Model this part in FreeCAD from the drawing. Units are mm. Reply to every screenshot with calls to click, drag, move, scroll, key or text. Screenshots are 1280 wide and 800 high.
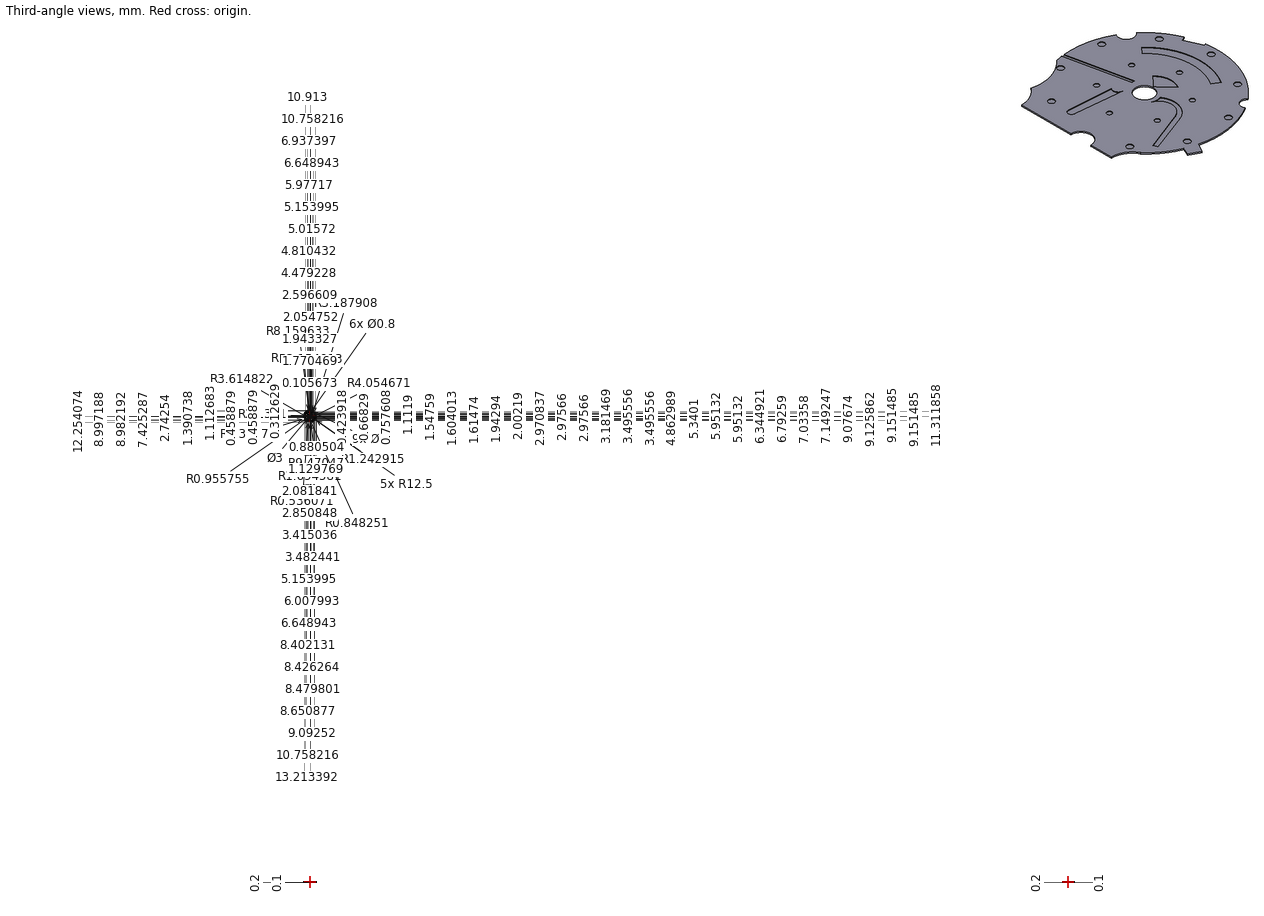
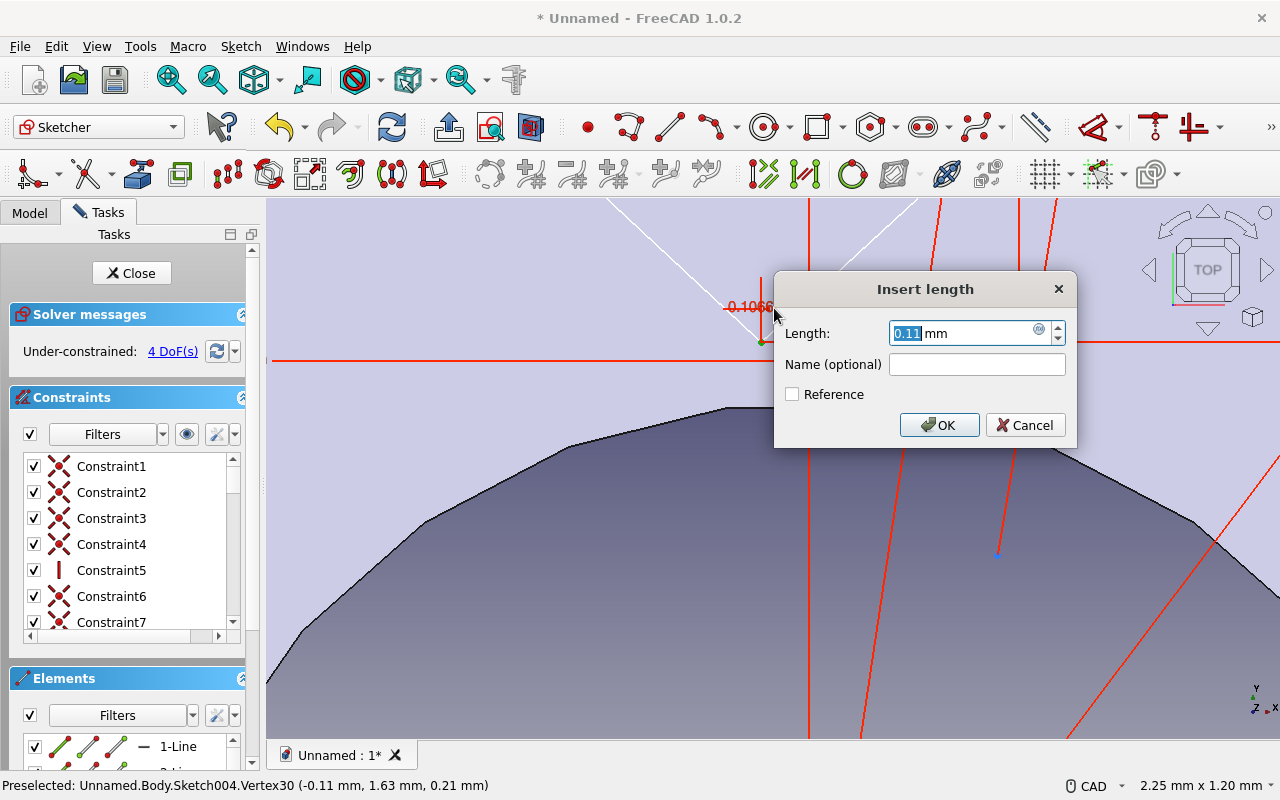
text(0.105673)
key(Return)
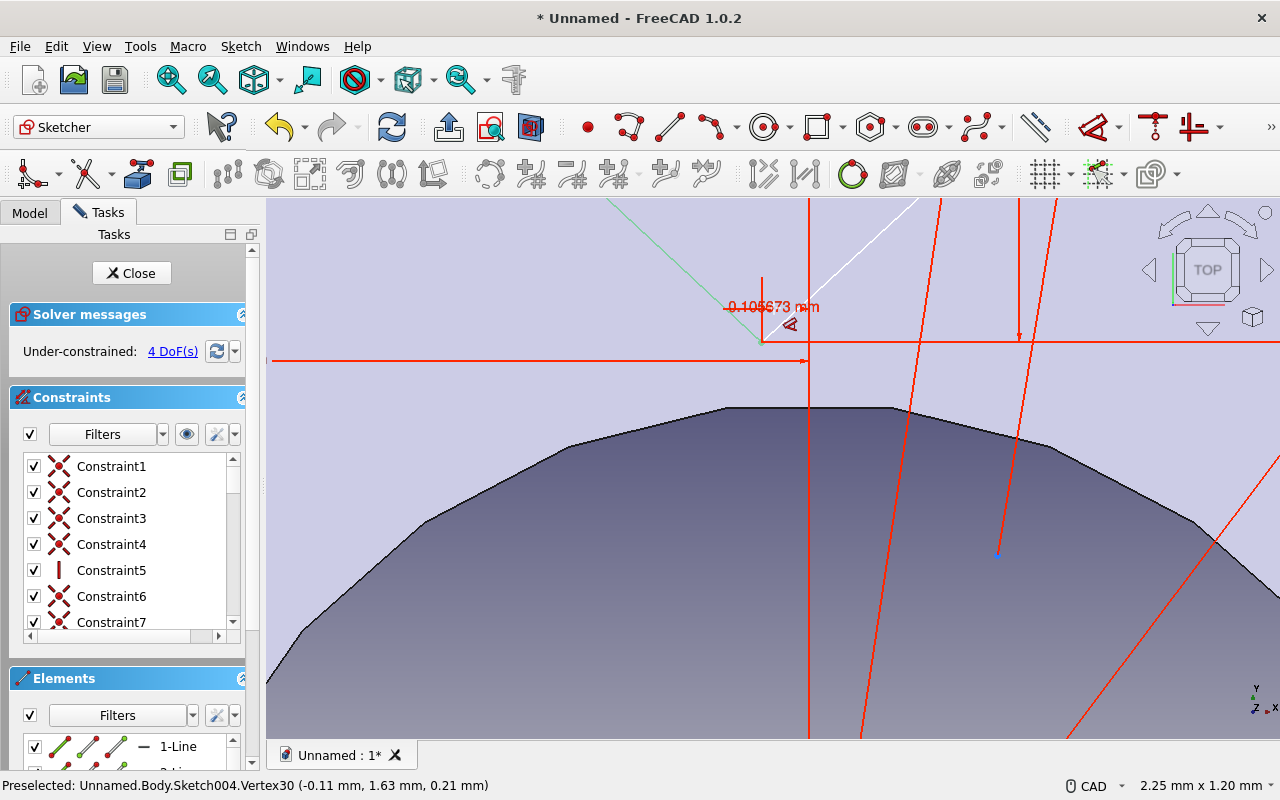
scroll(748, 434, down, 15)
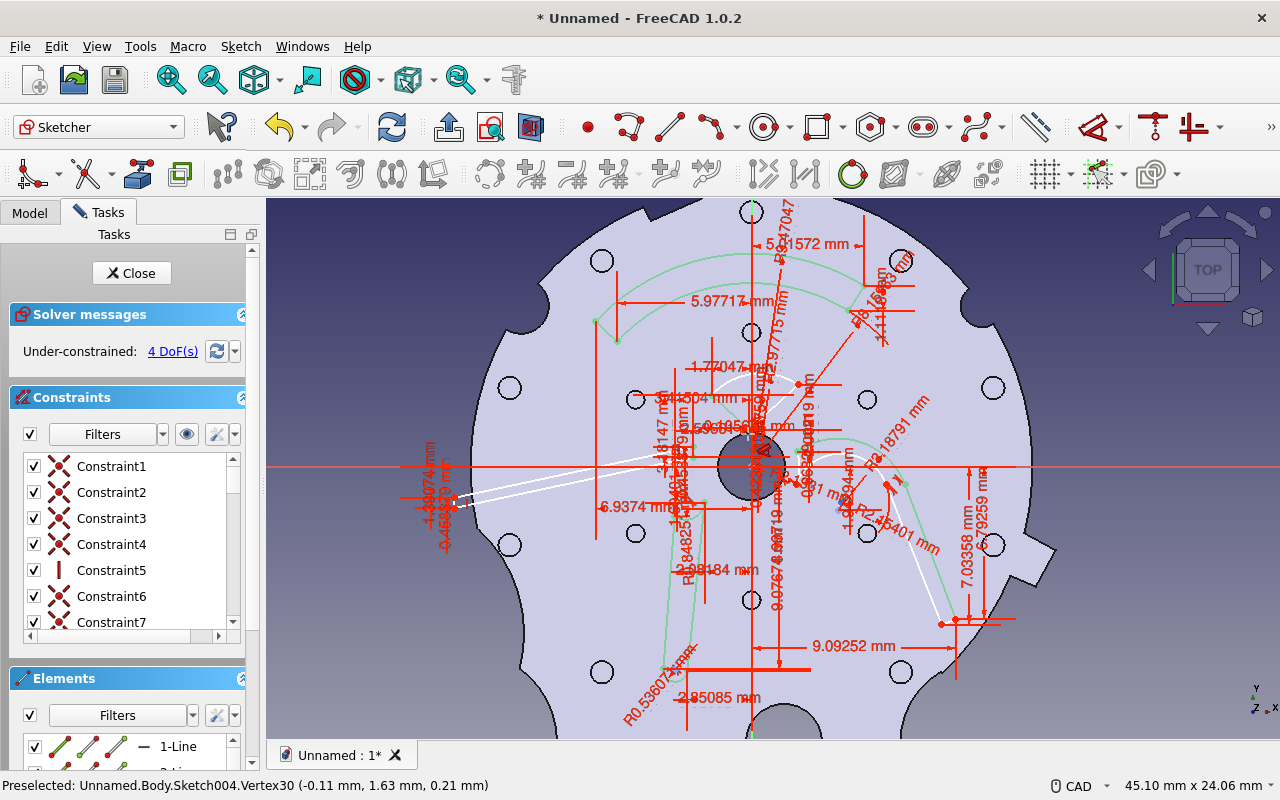
click(798, 385)
click(775, 549)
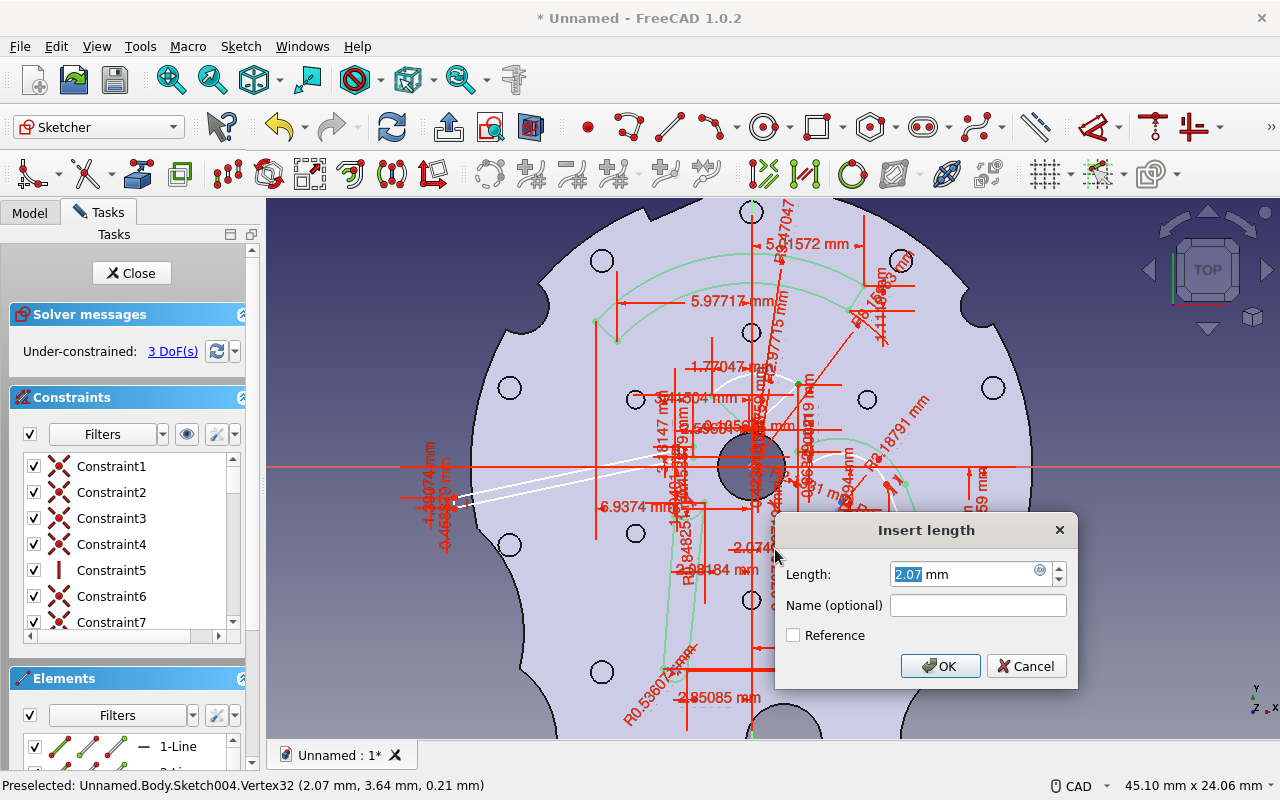
text(2.054752)
key(Return)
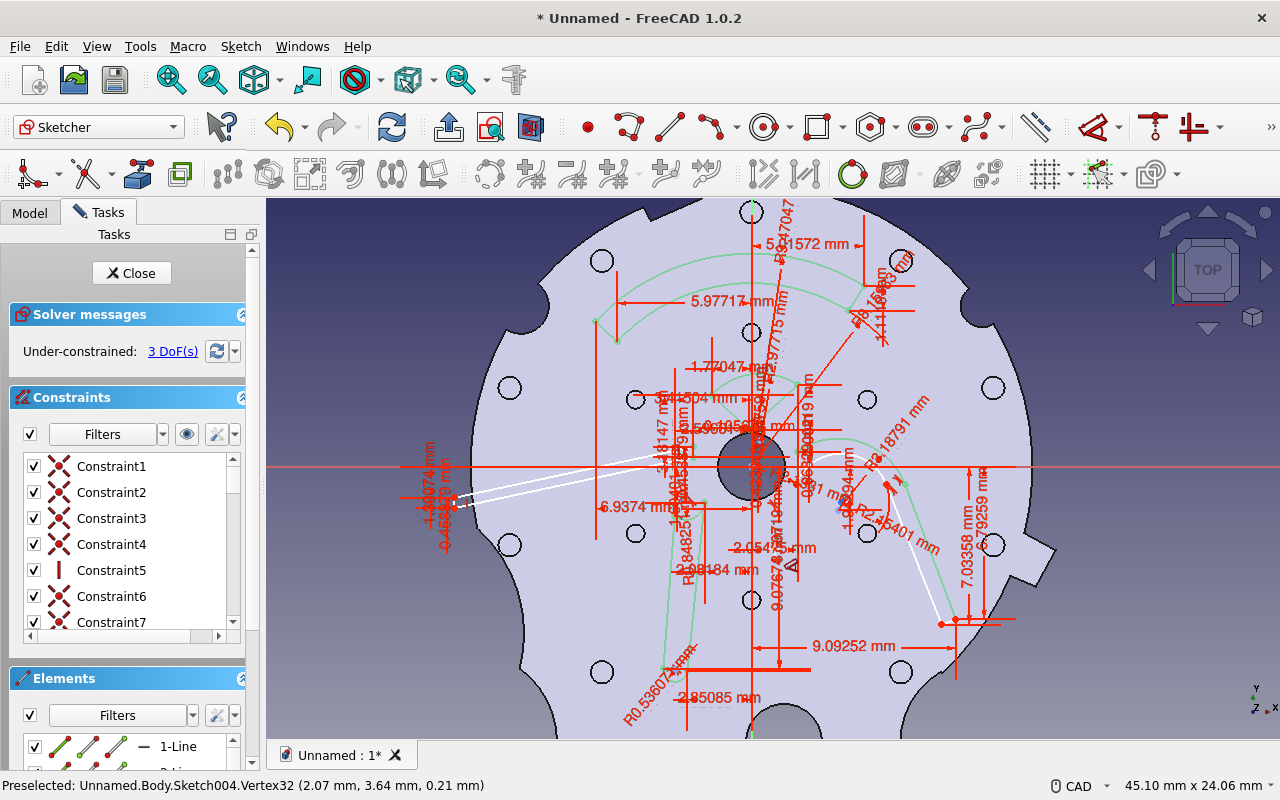
click(886, 484)
click(850, 566)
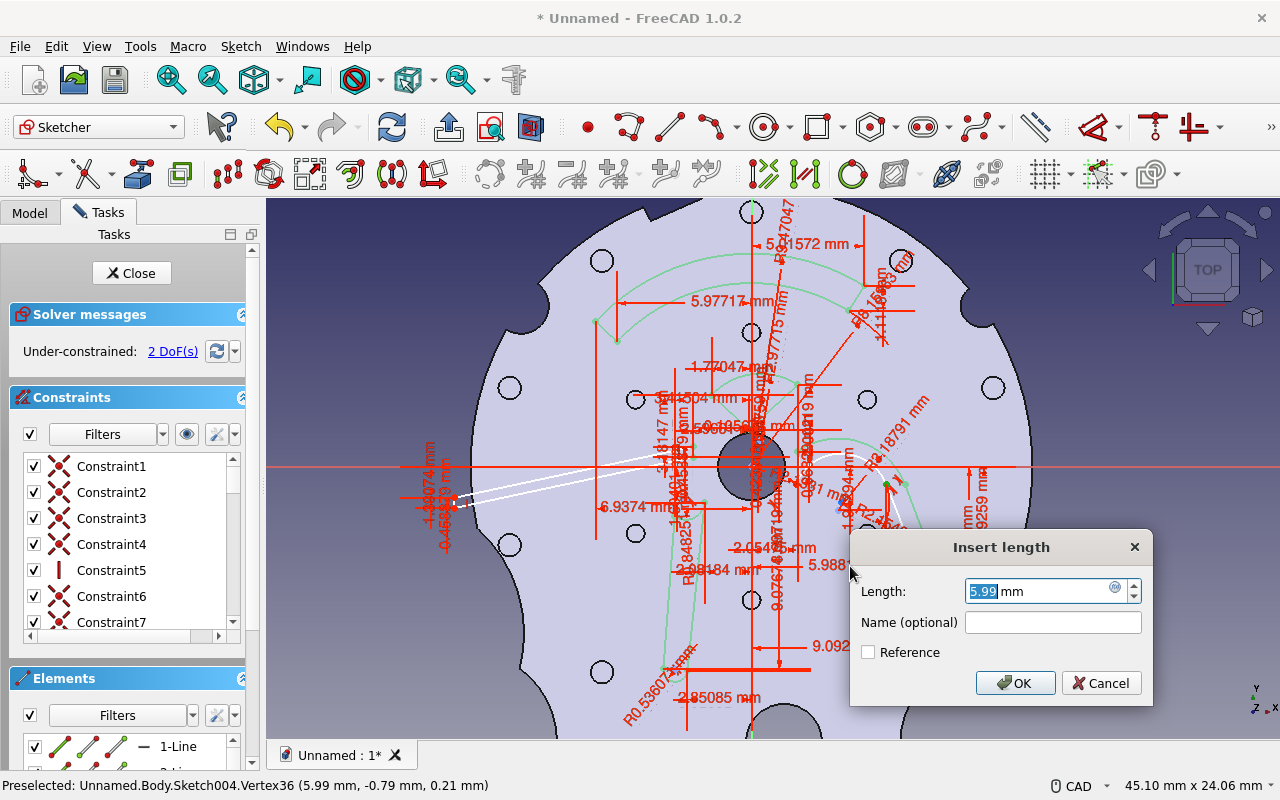
text(6.007993)
key(Return)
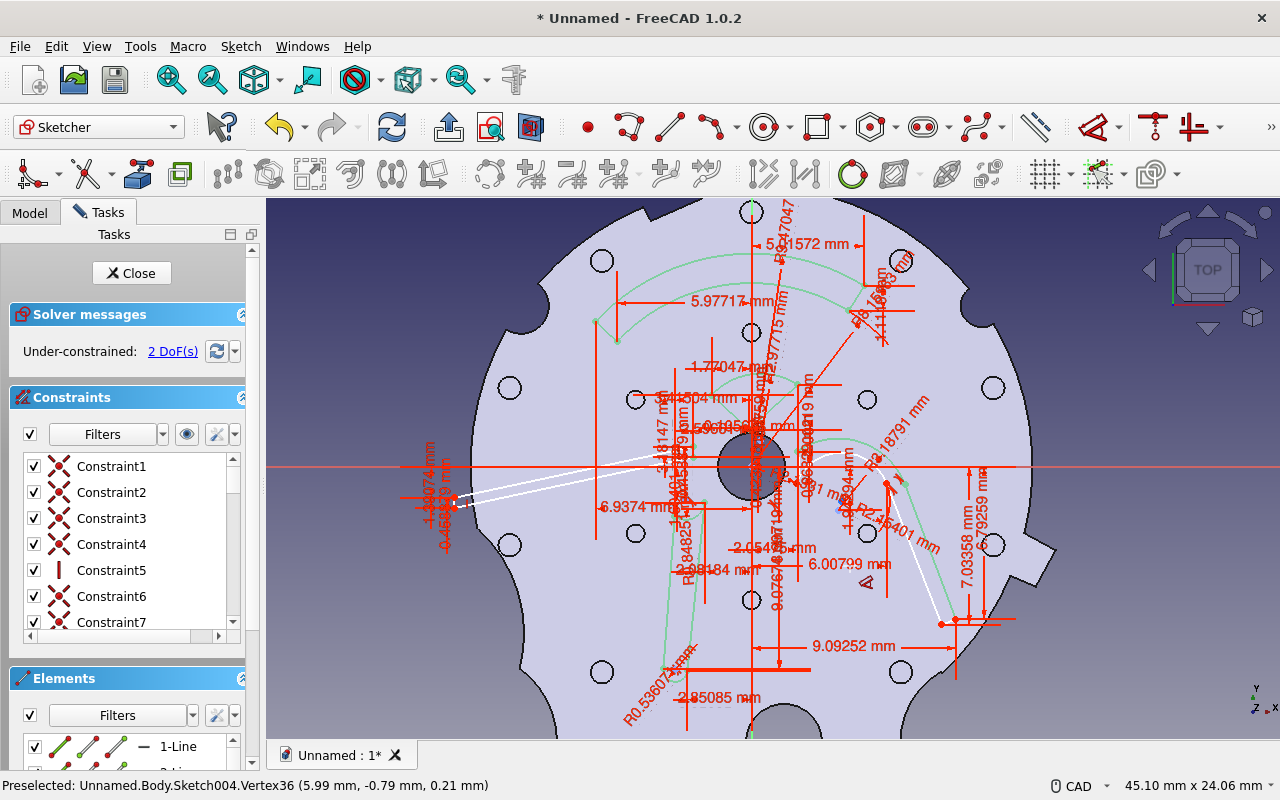
scroll(887, 484, up, 5)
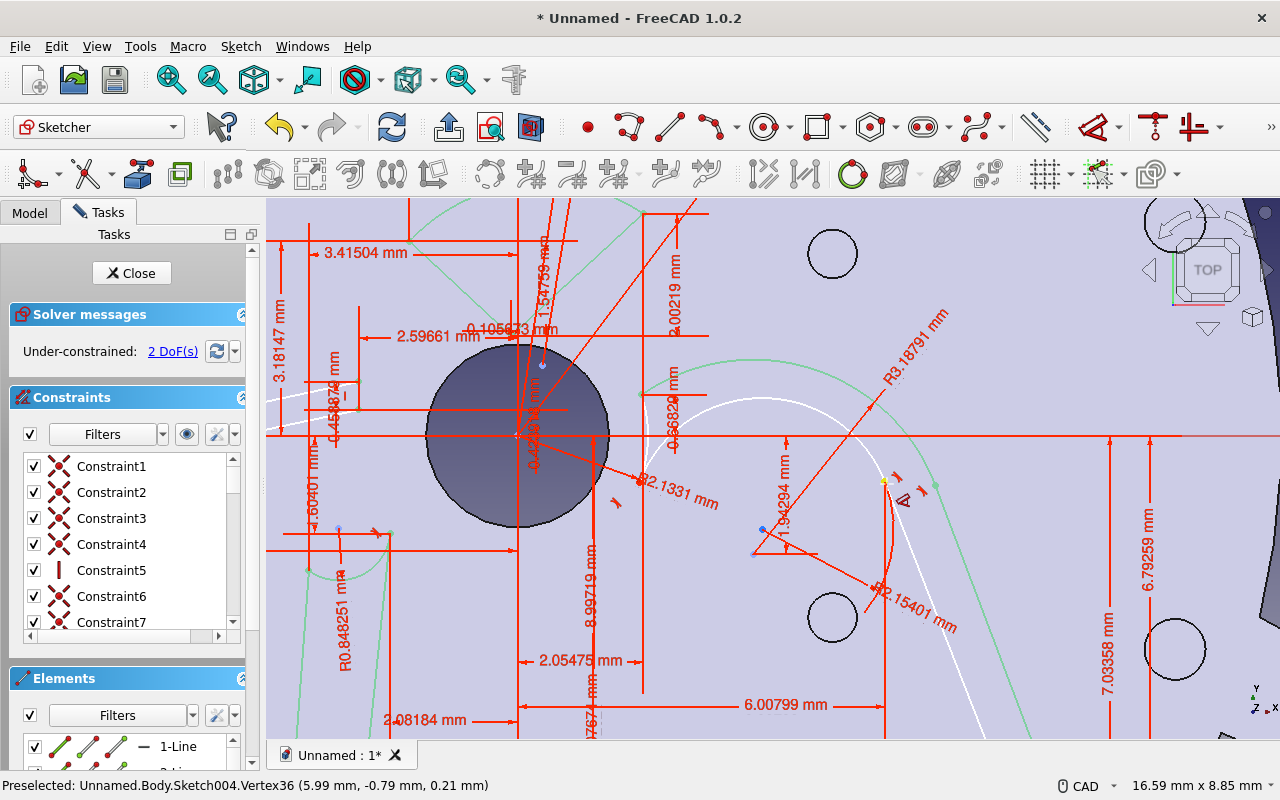
click(885, 482)
click(484, 459)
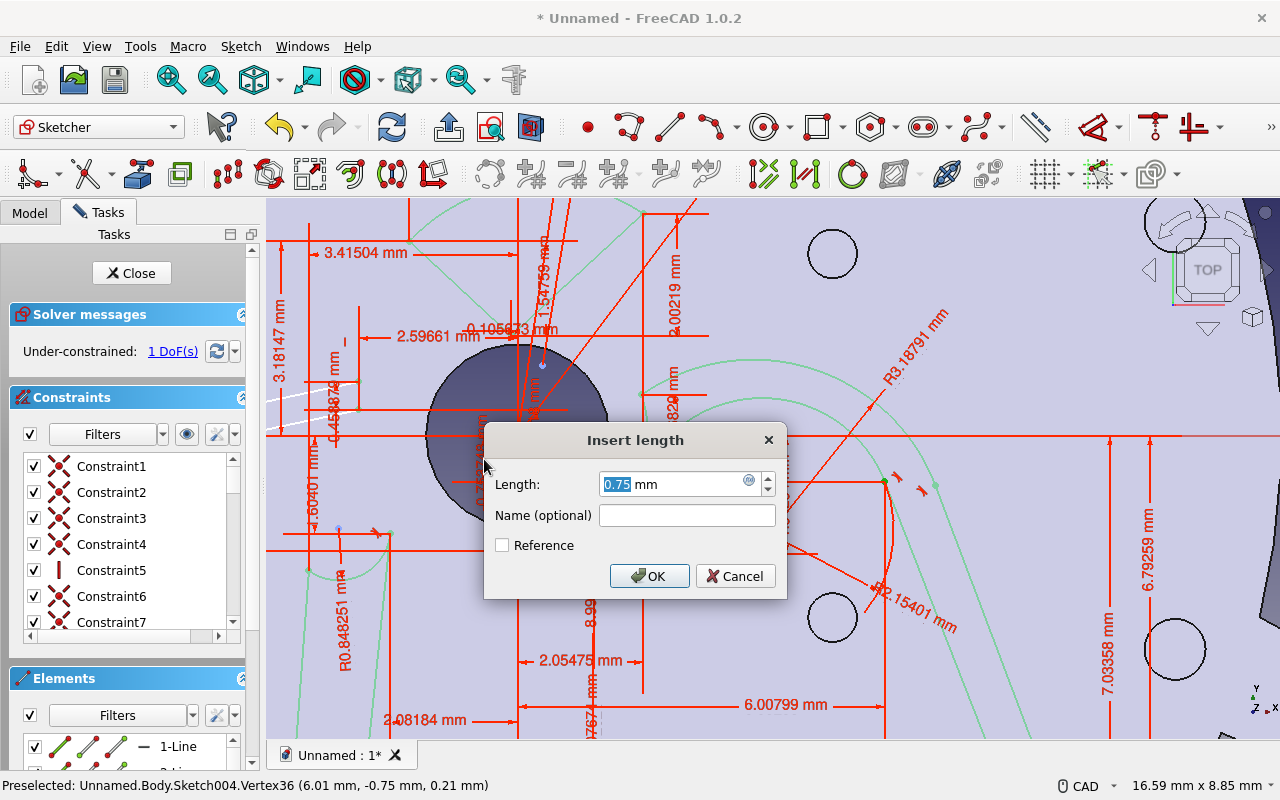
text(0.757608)
key(Return)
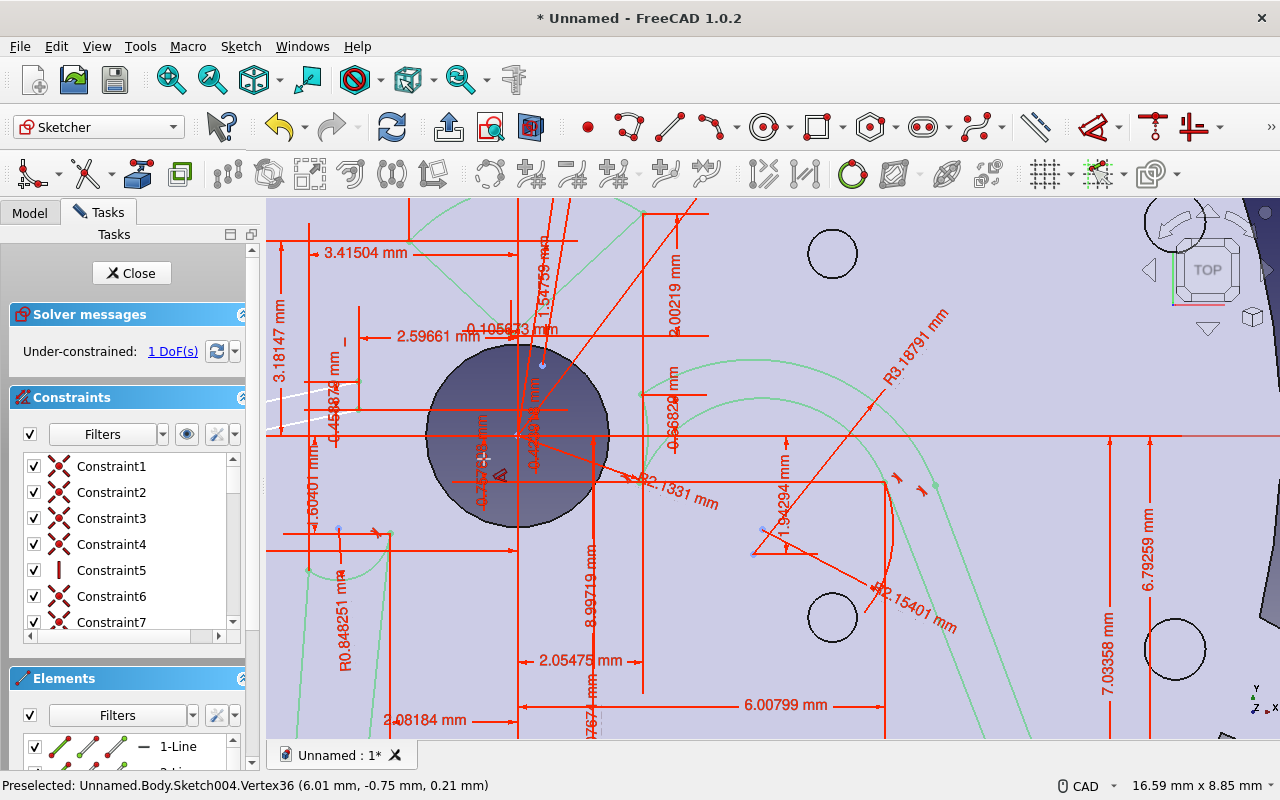
scroll(839, 480, down, 6)